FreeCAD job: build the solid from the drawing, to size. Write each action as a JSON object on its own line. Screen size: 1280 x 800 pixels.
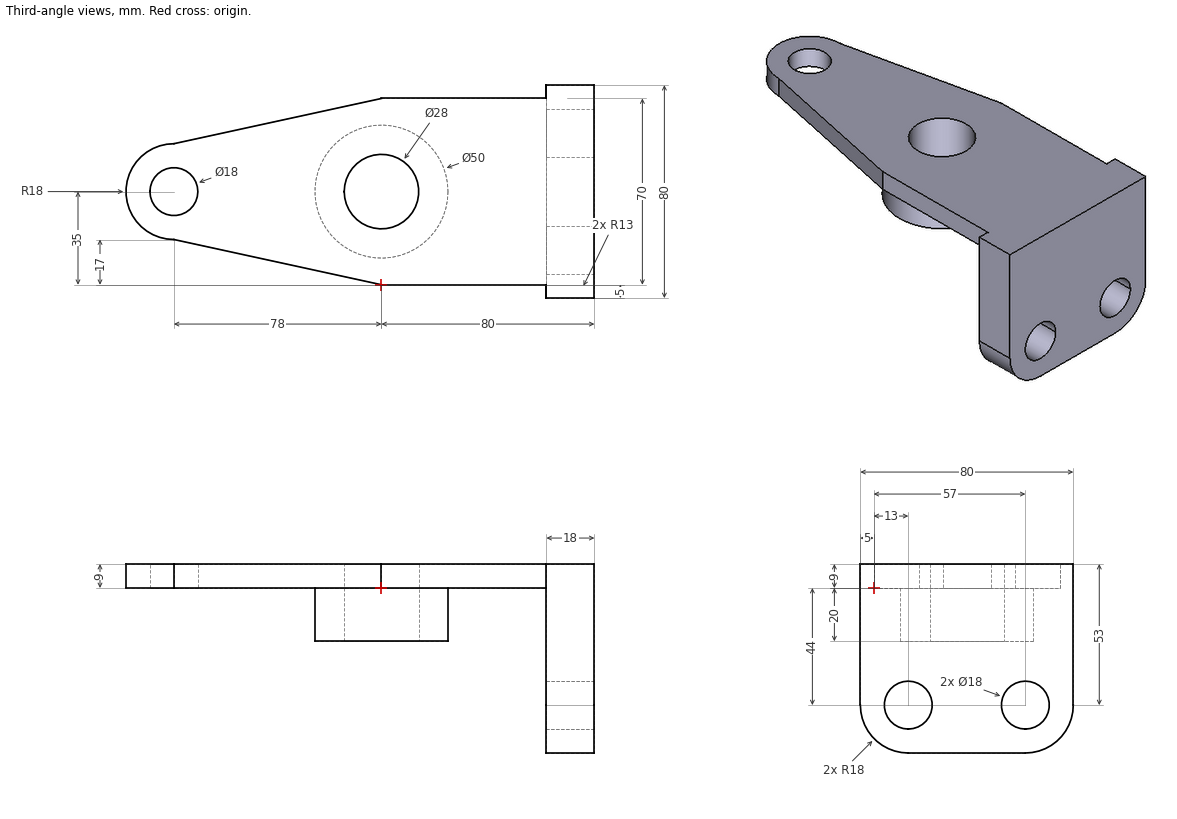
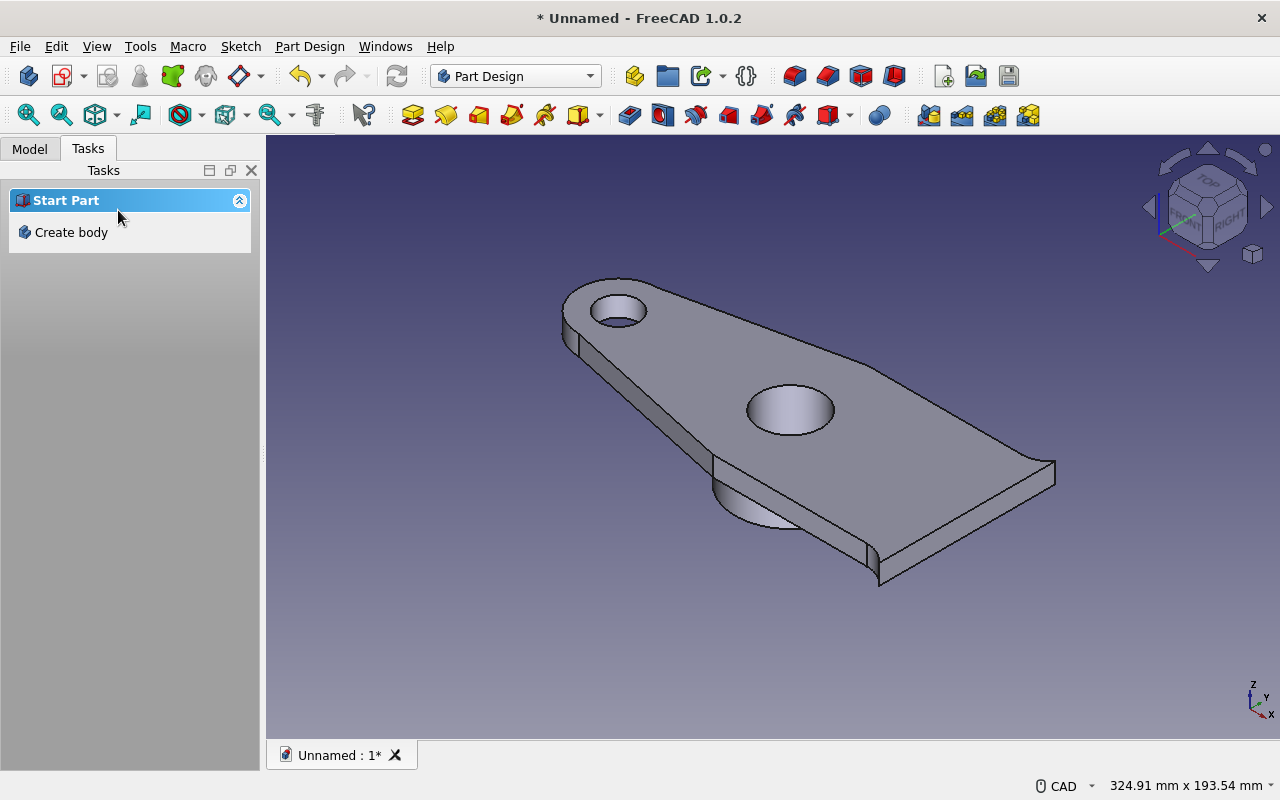
{"action": "left_click", "coordinate": [1043, 479]}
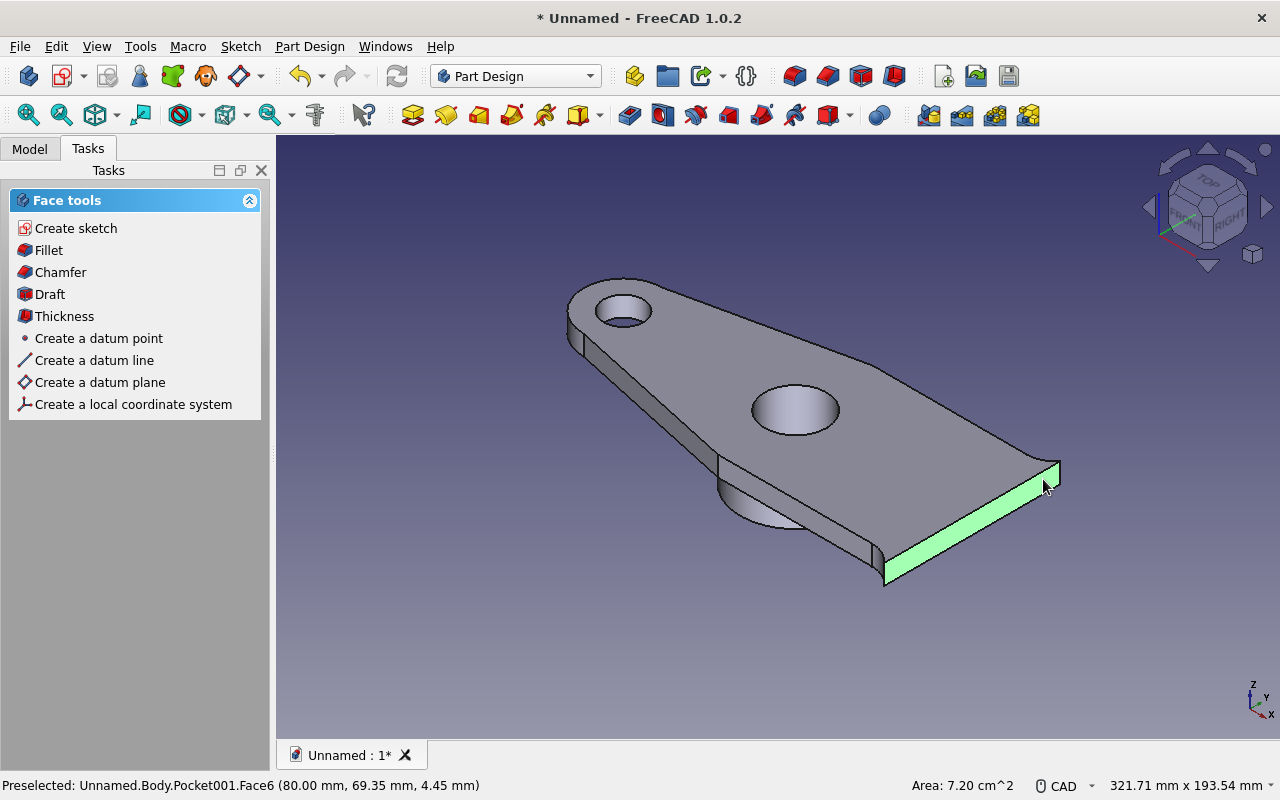
{"action": "left_click", "coordinate": [62, 76]}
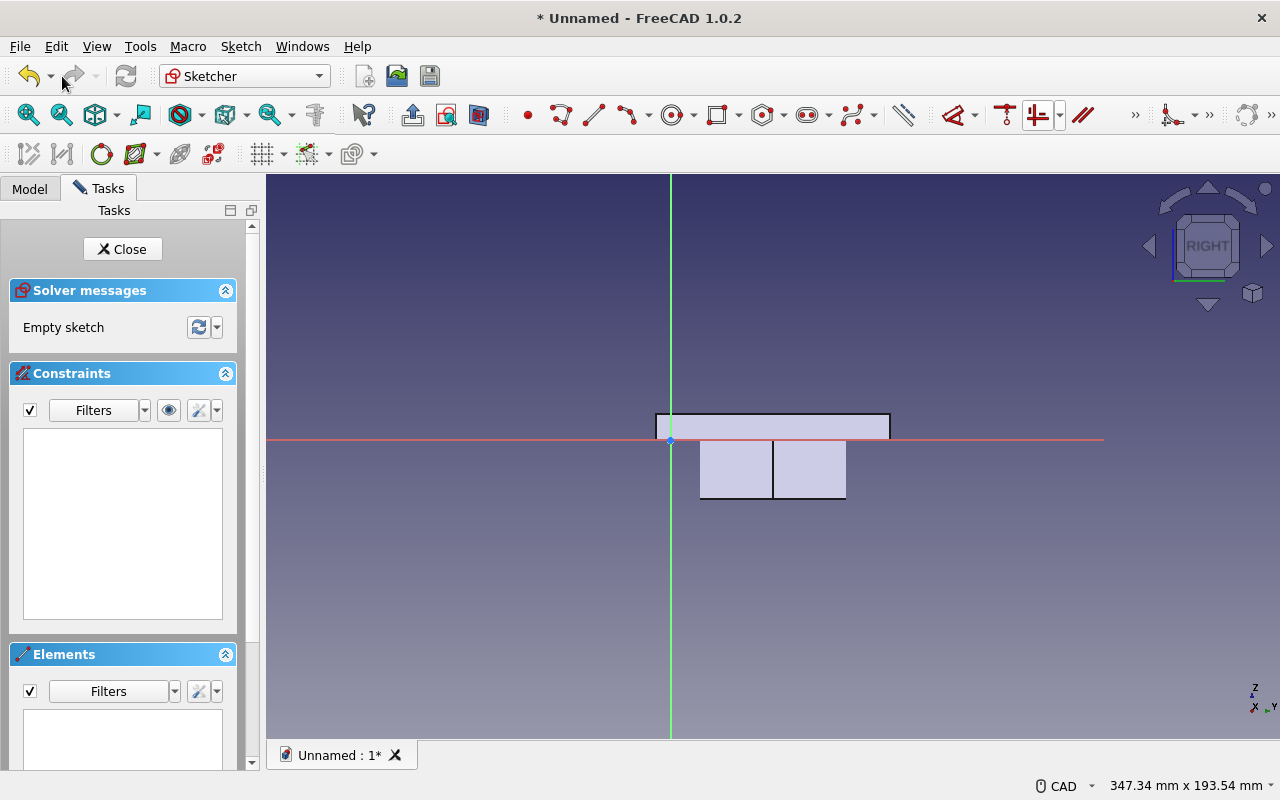
{"action": "scroll", "coordinate": [856, 592], "scroll_direction": "up", "scroll_amount": 3}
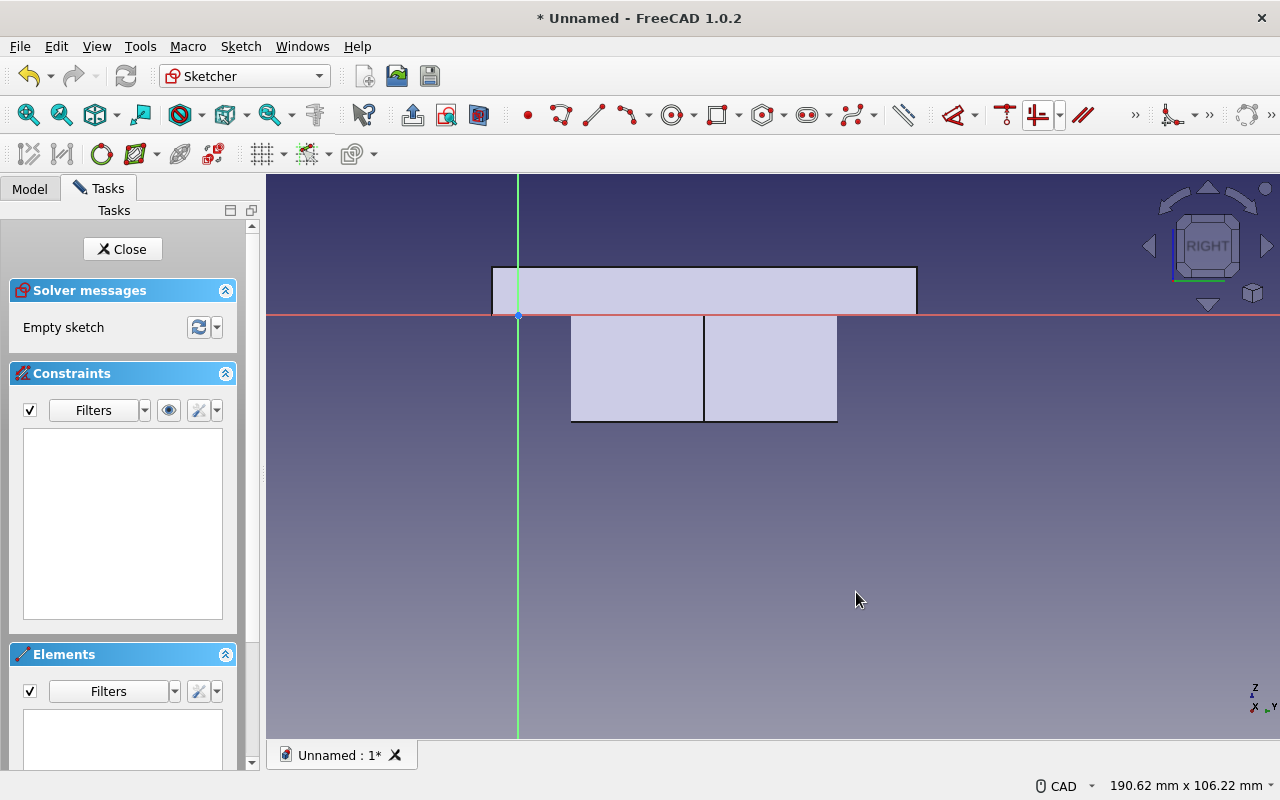
{"action": "left_click", "coordinate": [561, 116]}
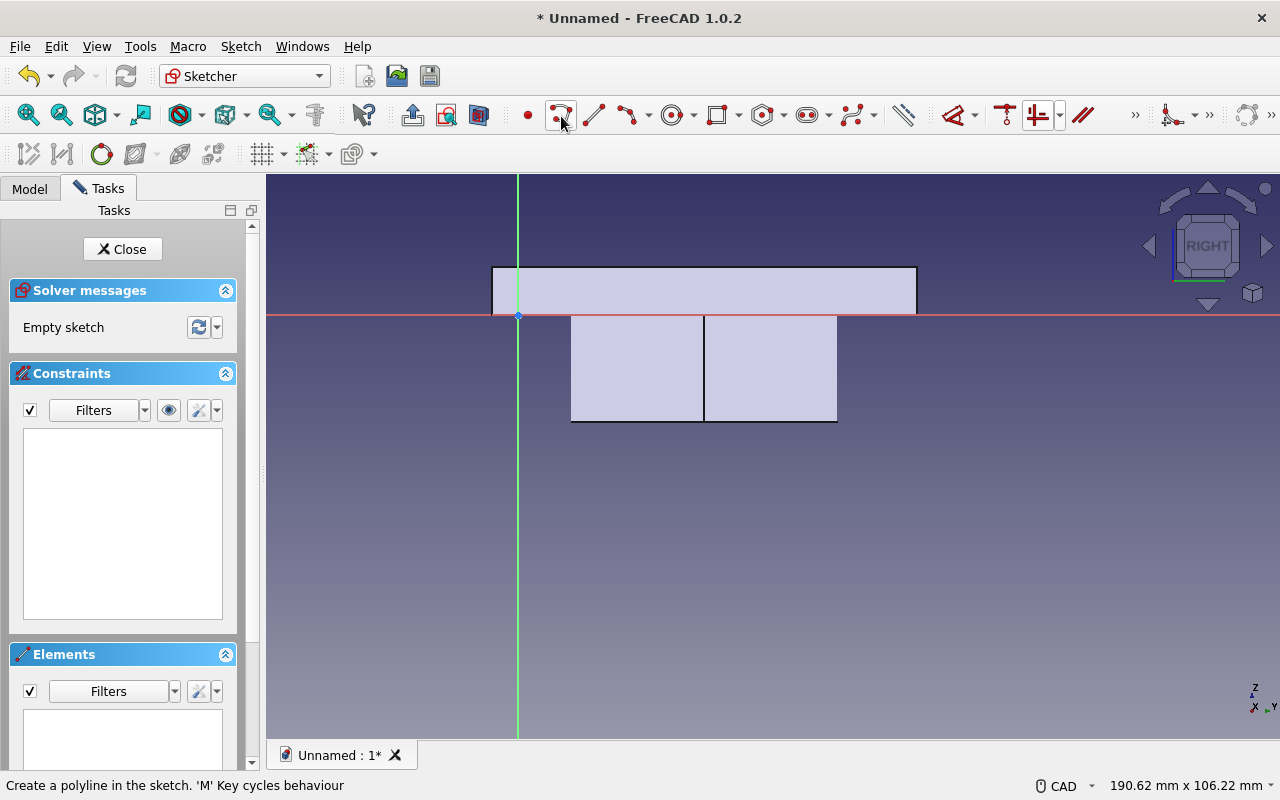
{"action": "left_click", "coordinate": [917, 549]}
{"action": "left_click", "coordinate": [917, 267]}
{"action": "left_click", "coordinate": [492, 267]}
{"action": "left_click", "coordinate": [492, 549]}
{"action": "right_click", "coordinate": [492, 549]}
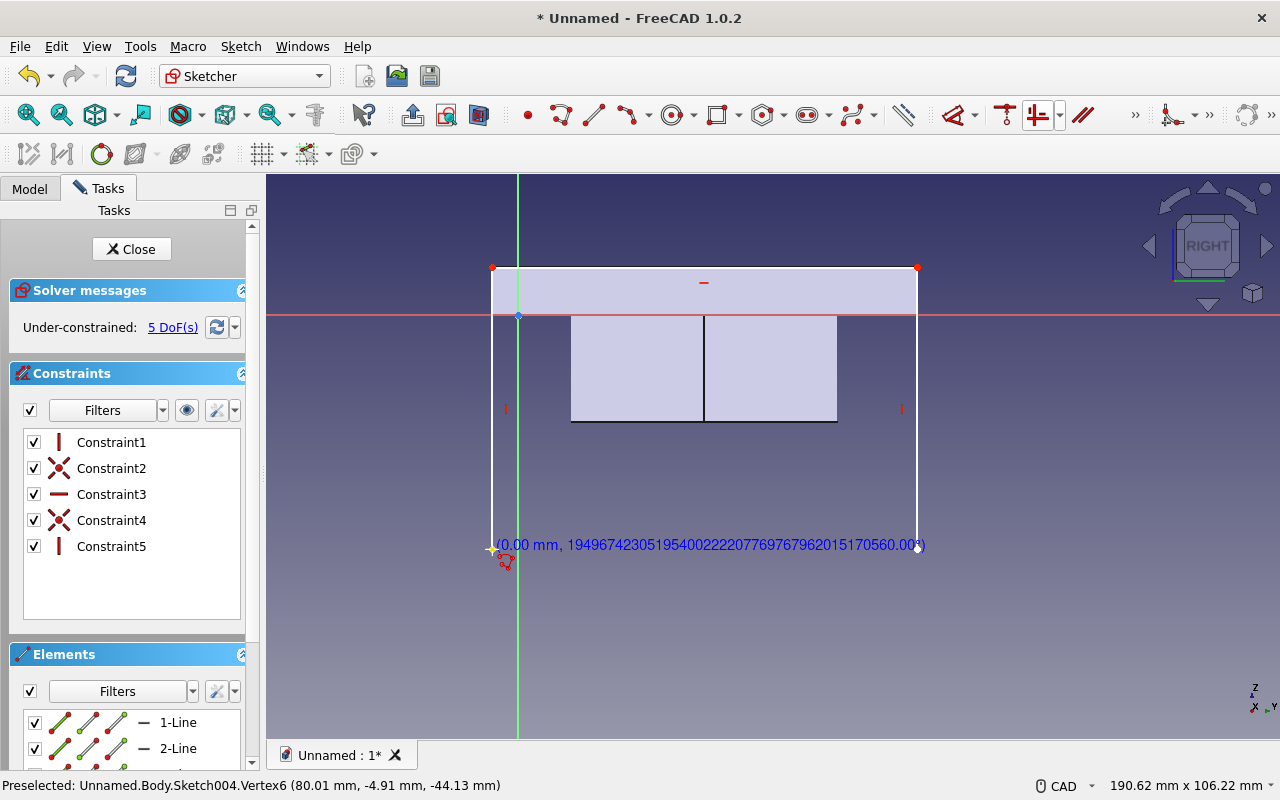
{"action": "left_click", "coordinate": [594, 116]}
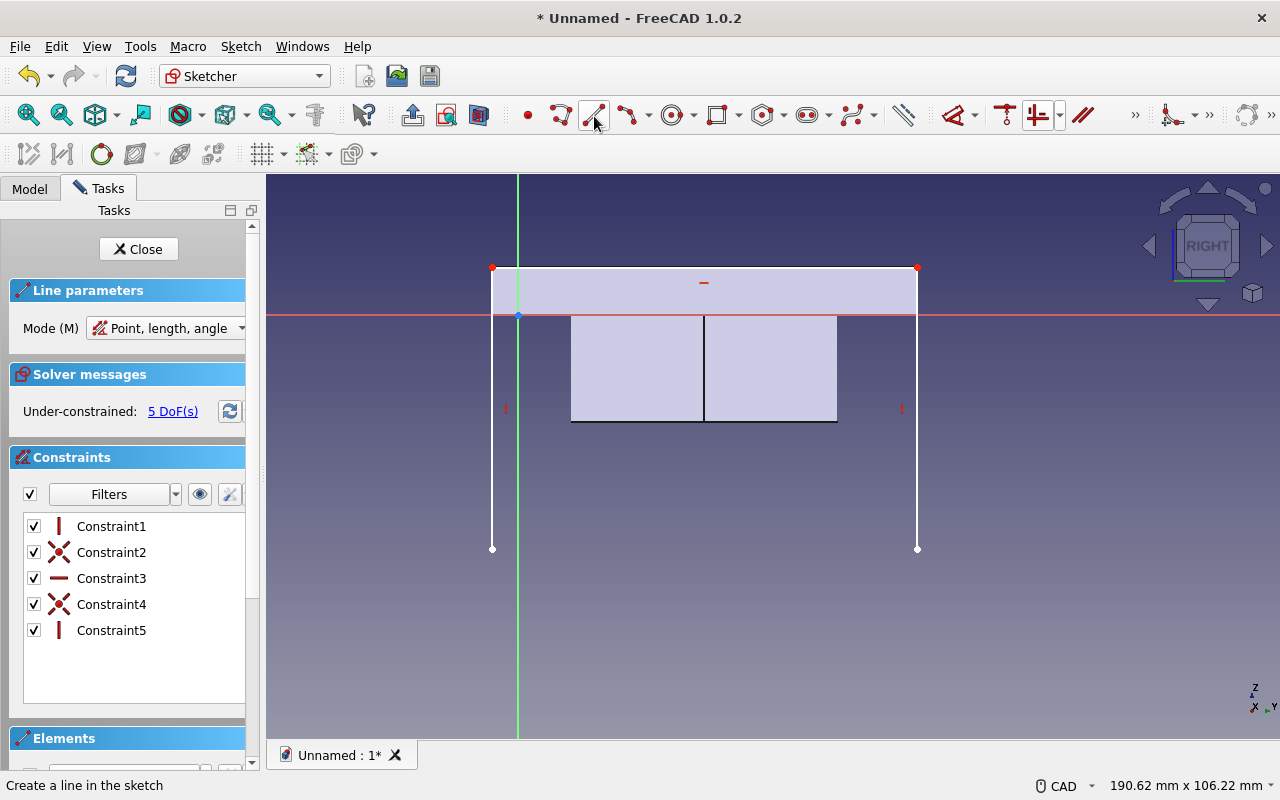
{"action": "left_click", "coordinate": [587, 645]}
{"action": "left_click", "coordinate": [821, 645]}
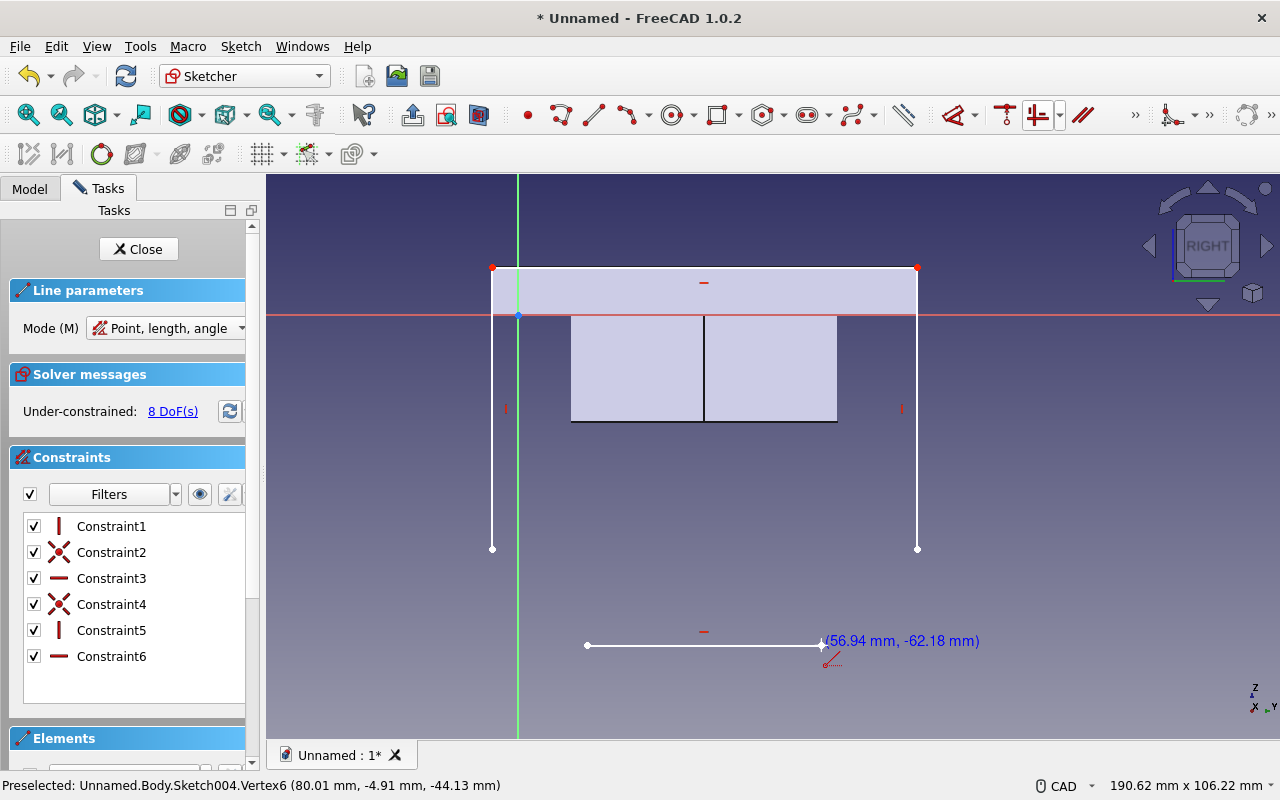
{"action": "left_click", "coordinate": [626, 116]}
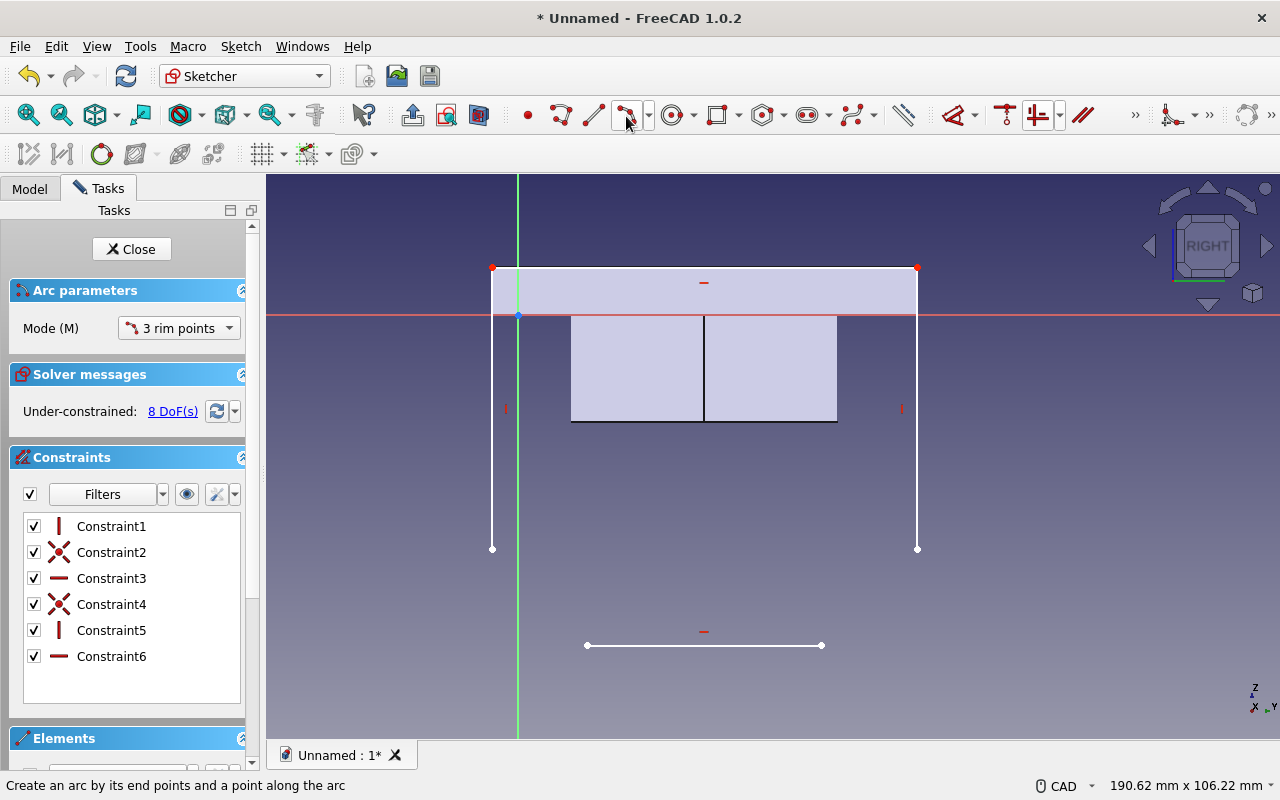
{"action": "left_click", "coordinate": [492, 550]}
{"action": "left_click", "coordinate": [587, 646]}
{"action": "left_click", "coordinate": [502, 593]}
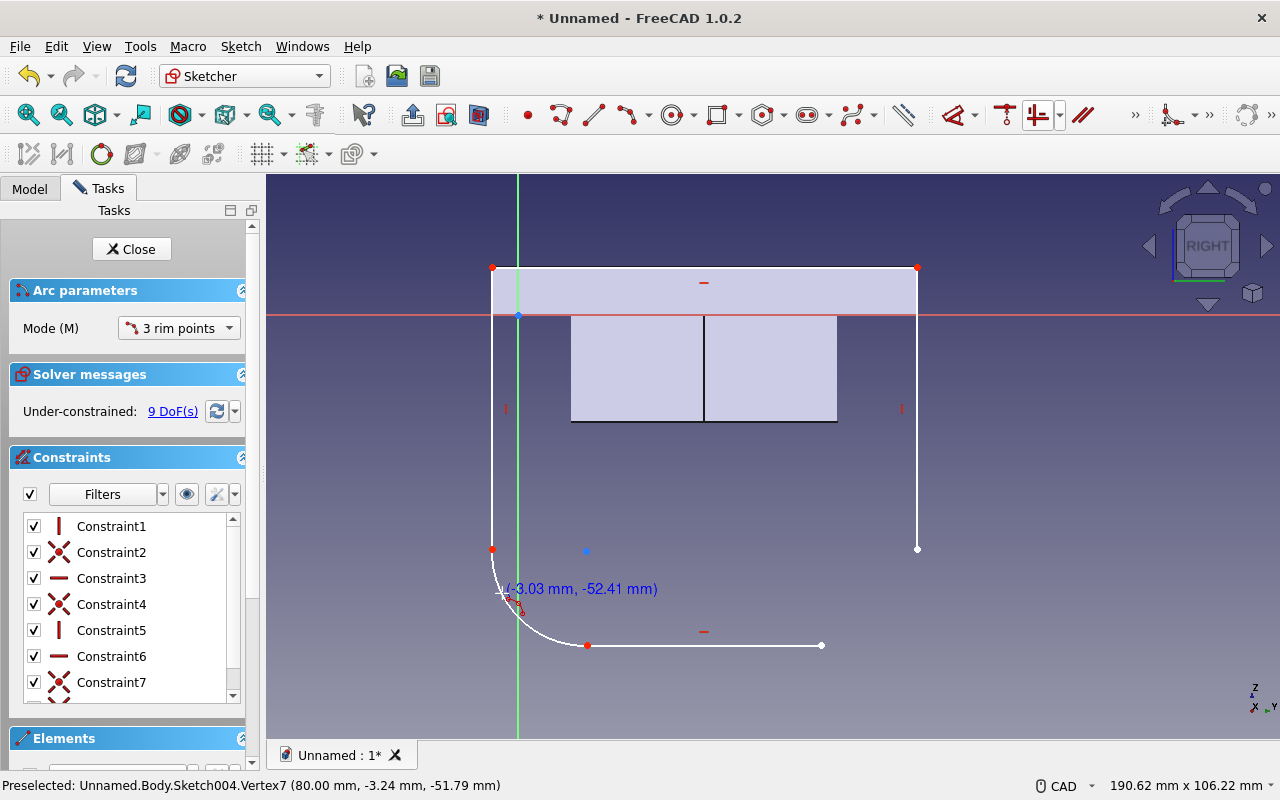
{"action": "left_click", "coordinate": [821, 646]}
{"action": "left_click", "coordinate": [917, 550]}
{"action": "left_click", "coordinate": [889, 617]}
{"action": "key", "text": "Escape"}